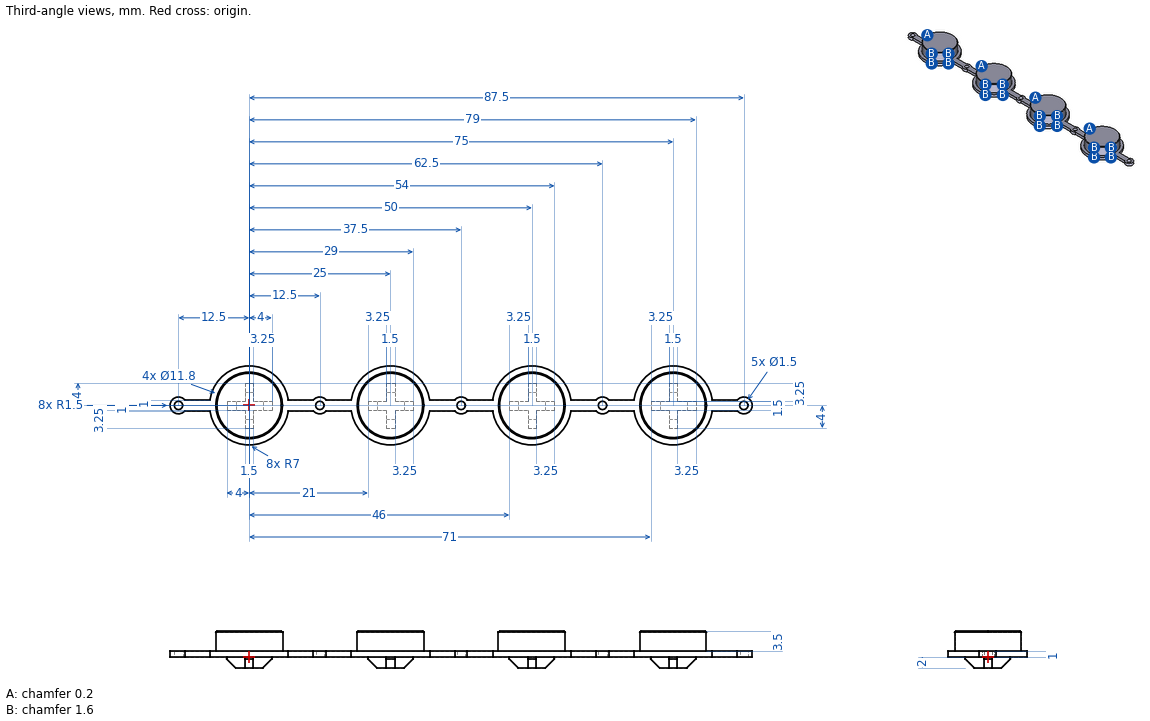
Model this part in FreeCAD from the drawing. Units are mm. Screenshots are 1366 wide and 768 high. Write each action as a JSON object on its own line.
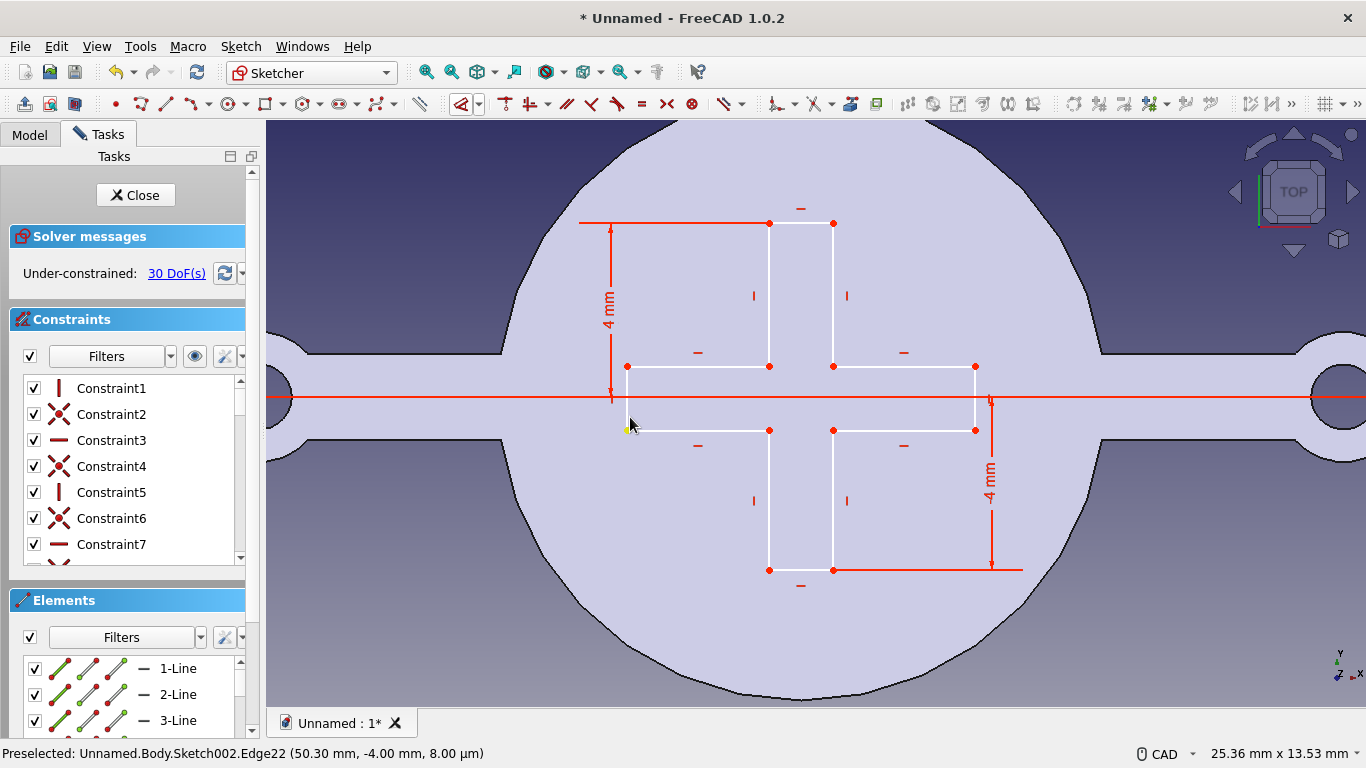
{"action": "left_click", "coordinate": [627, 411]}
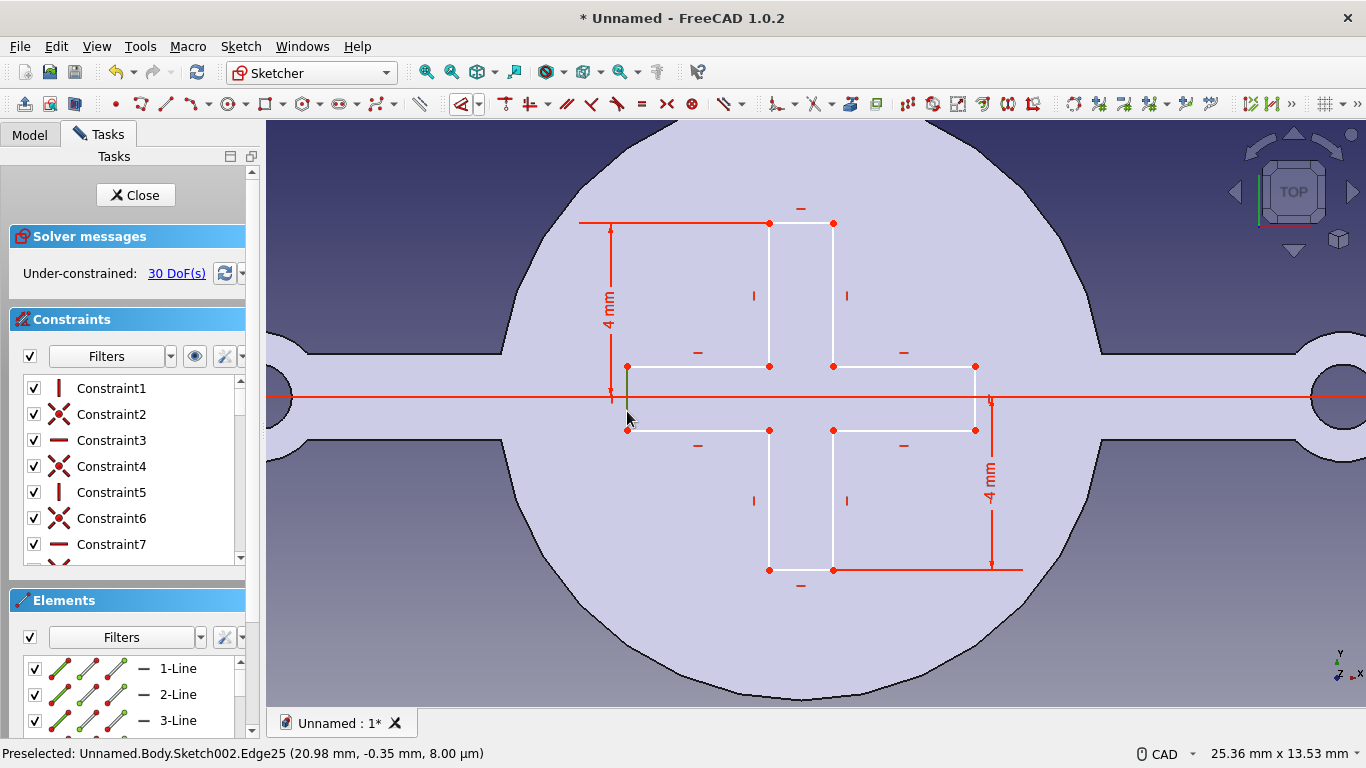
{"action": "key", "text": "i"}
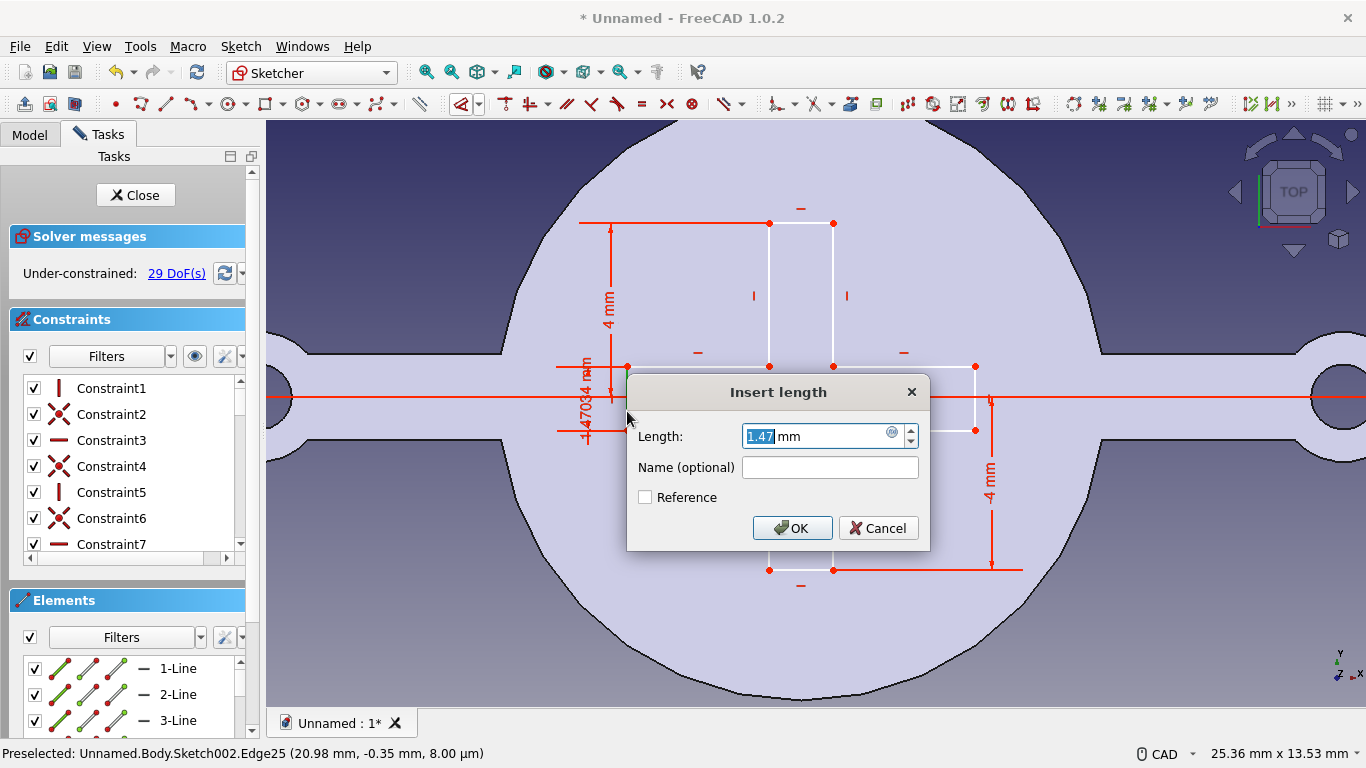
{"action": "type", "text": "1.5"}
{"action": "key", "text": "Return"}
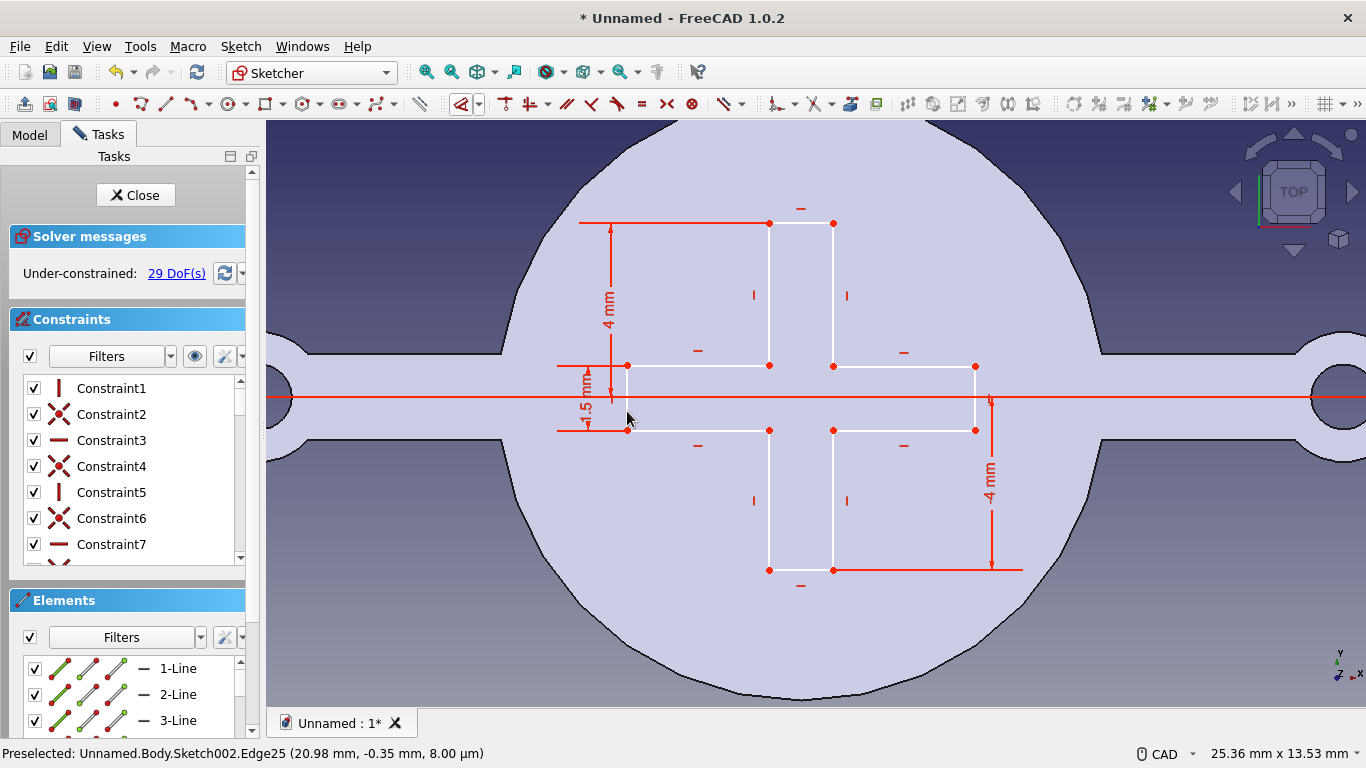
{"action": "left_click", "coordinate": [789, 223]}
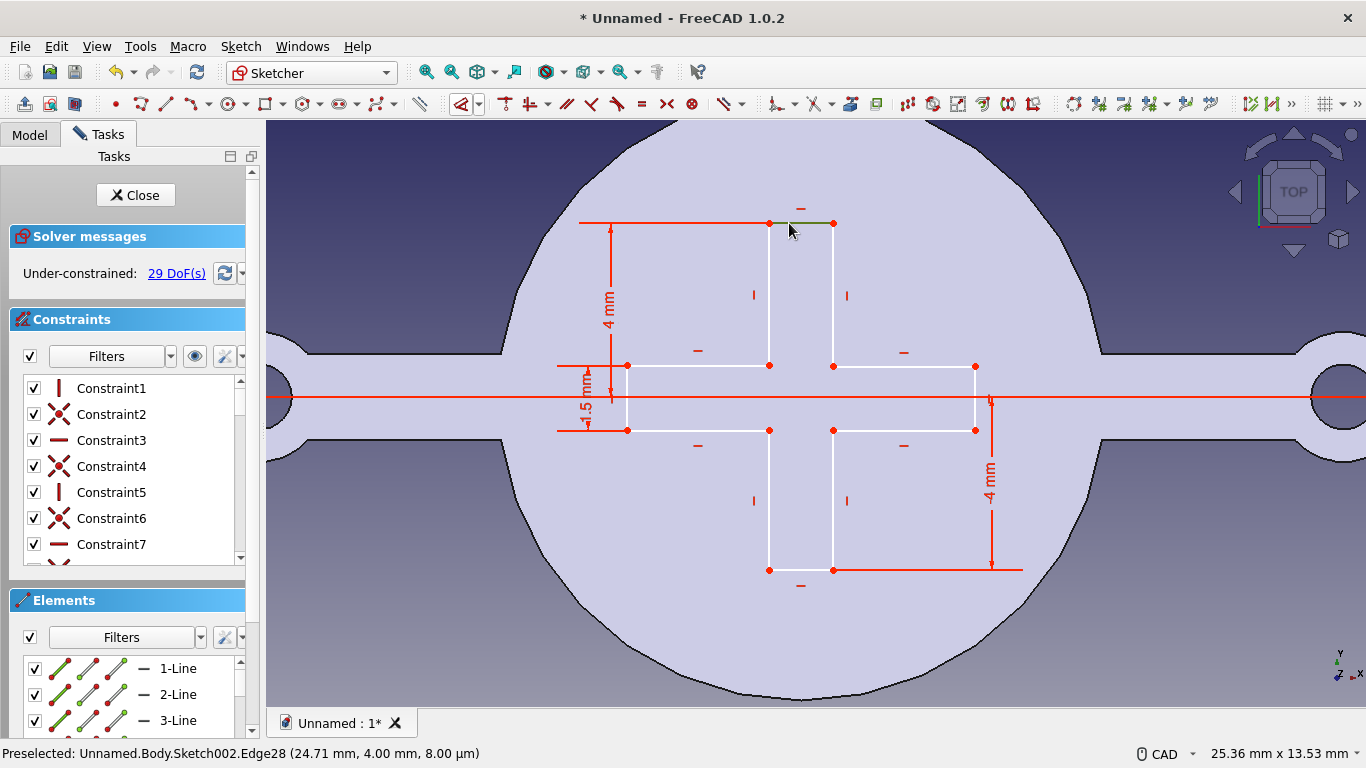
{"action": "left_click", "coordinate": [478, 104]}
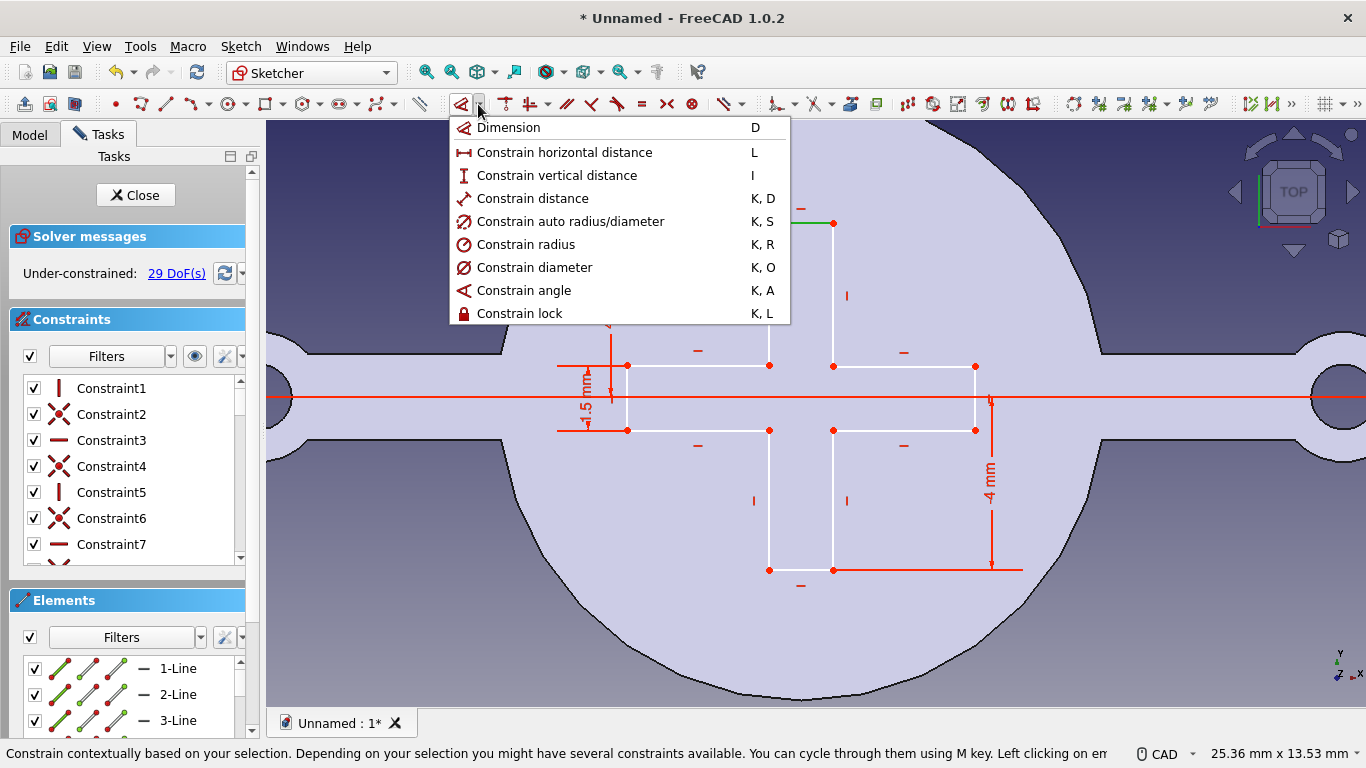
{"action": "left_click", "coordinate": [620, 152]}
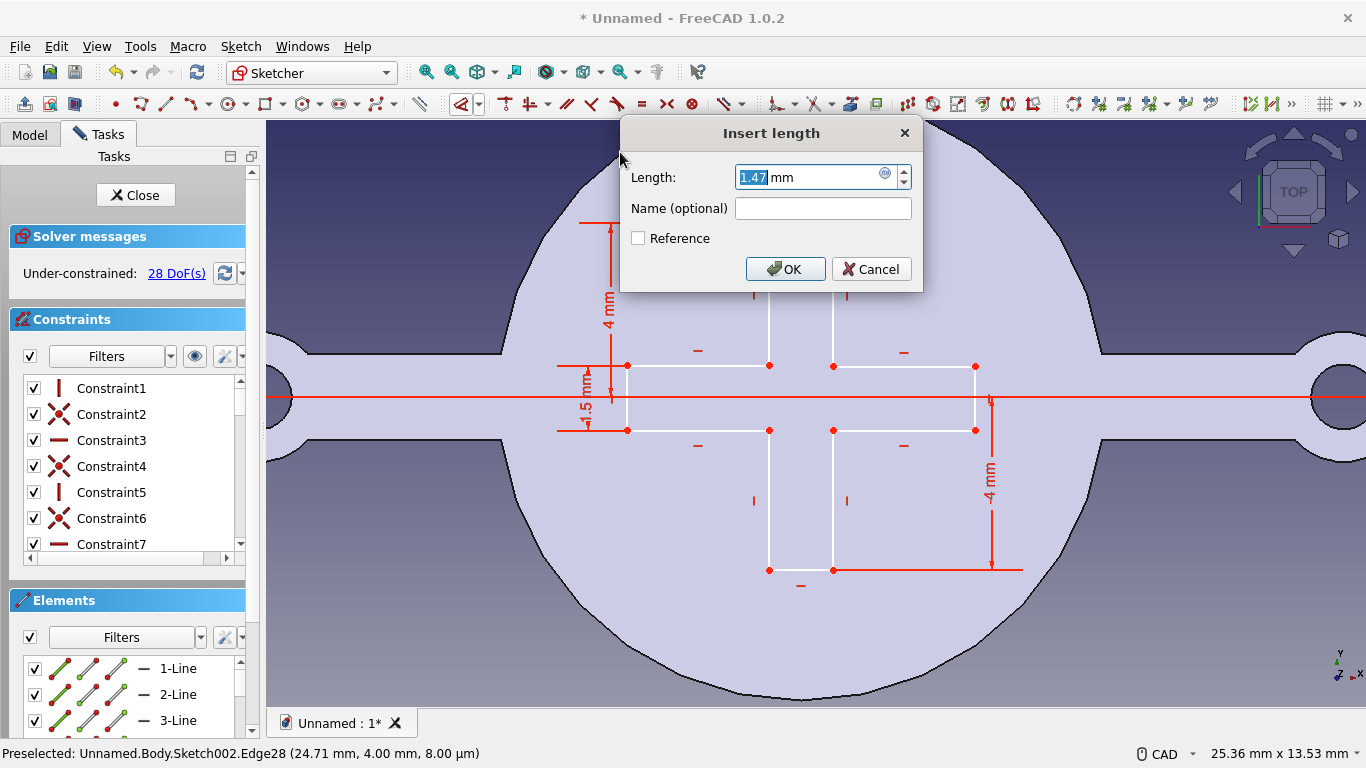
{"action": "type", "text": "1.5"}
{"action": "key", "text": "Return"}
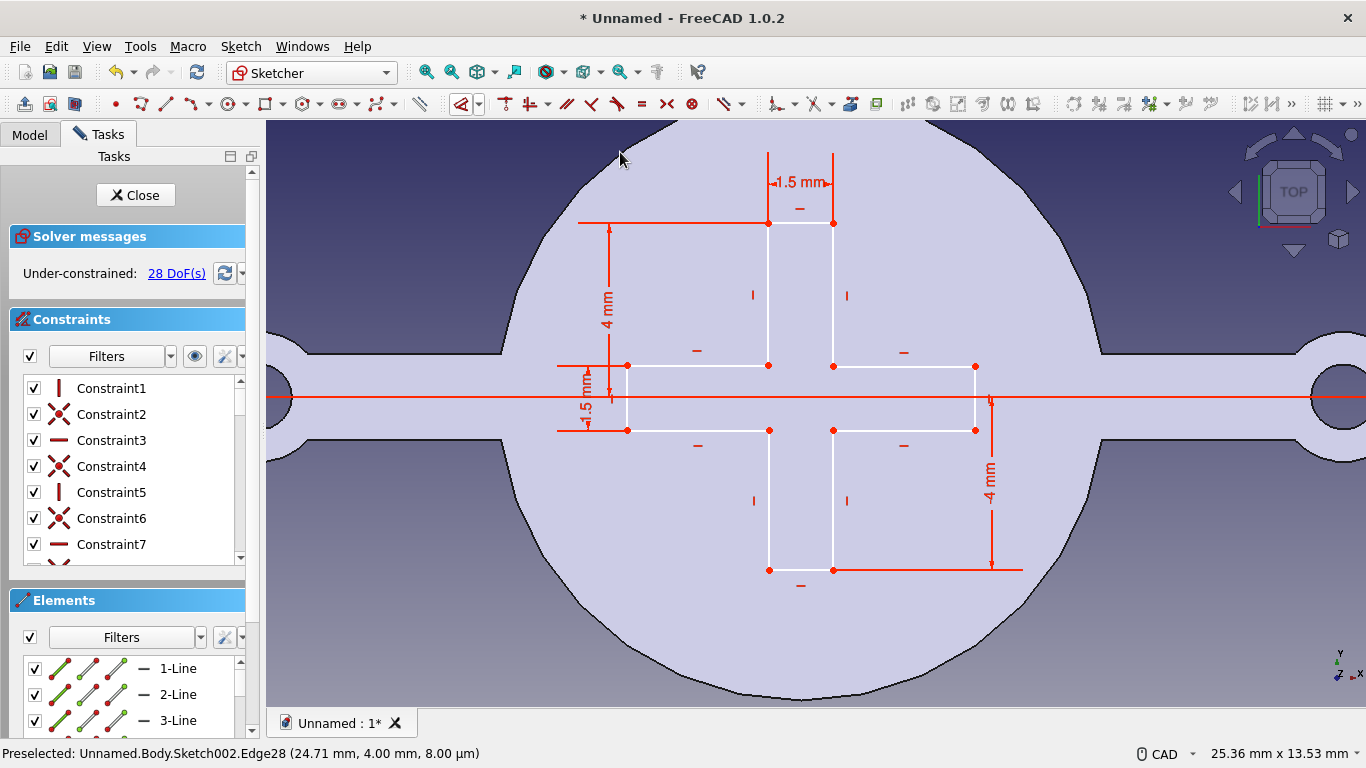
{"action": "scroll", "coordinate": [975, 386], "scroll_direction": "up", "scroll_amount": 2}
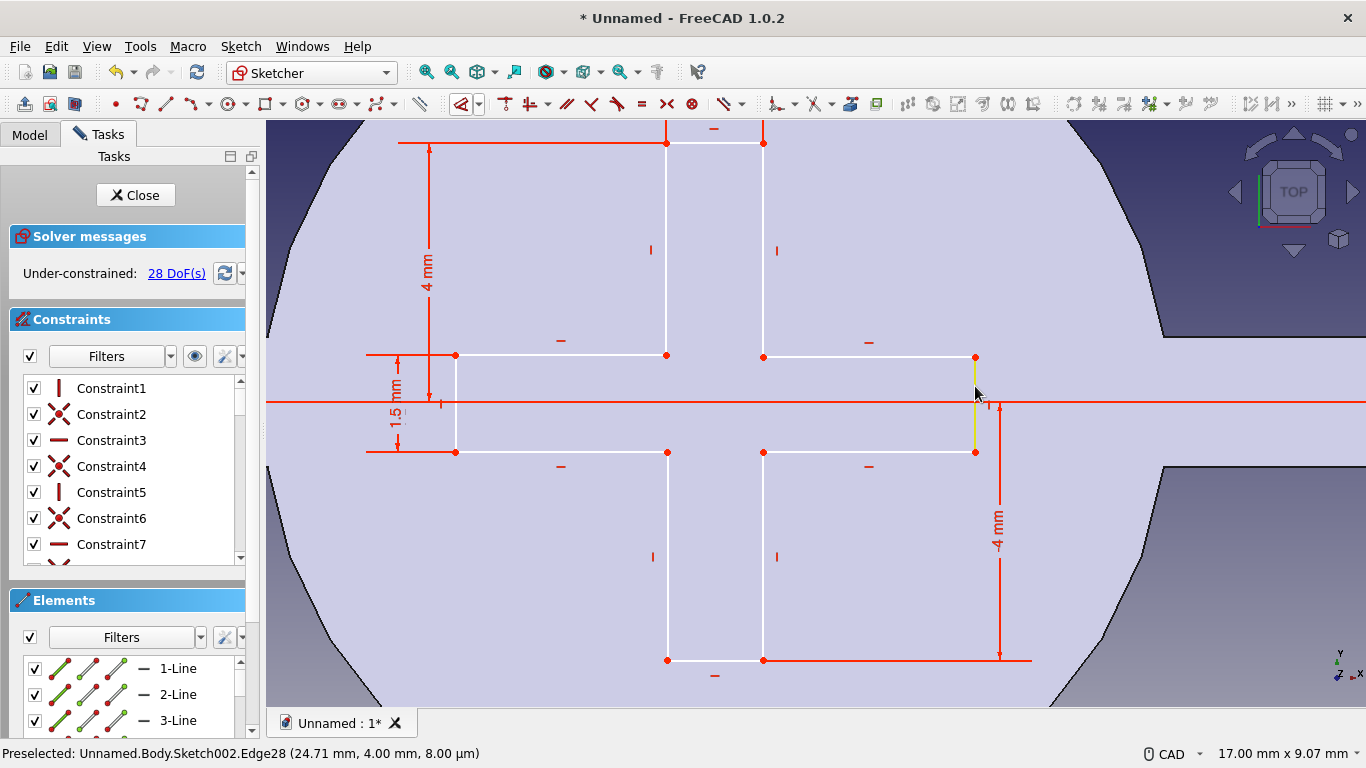
{"action": "left_click", "coordinate": [975, 386]}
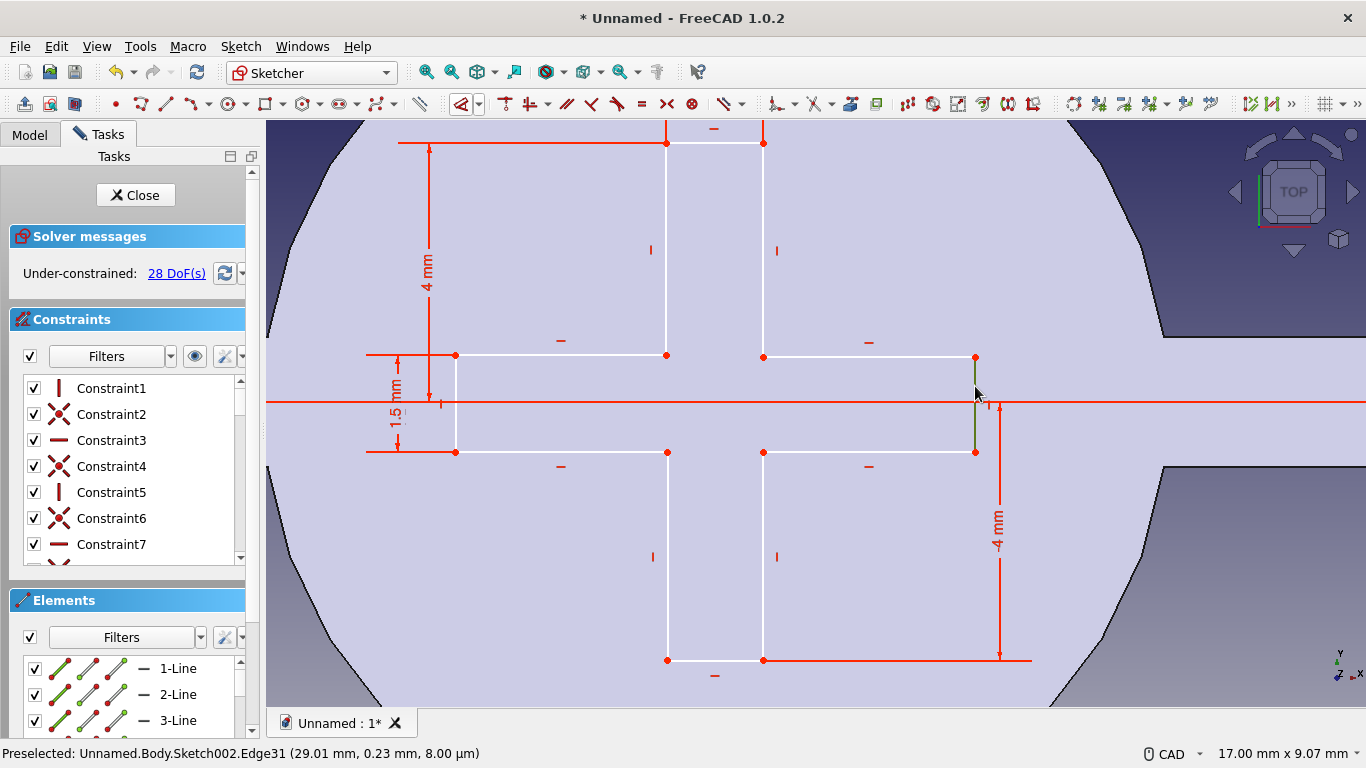
{"action": "key", "text": "i"}